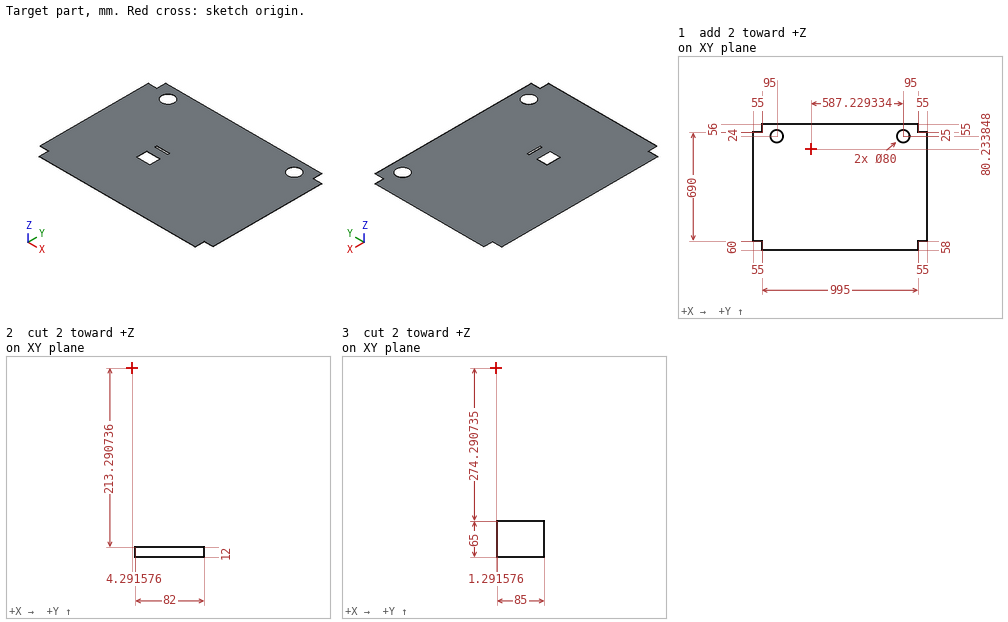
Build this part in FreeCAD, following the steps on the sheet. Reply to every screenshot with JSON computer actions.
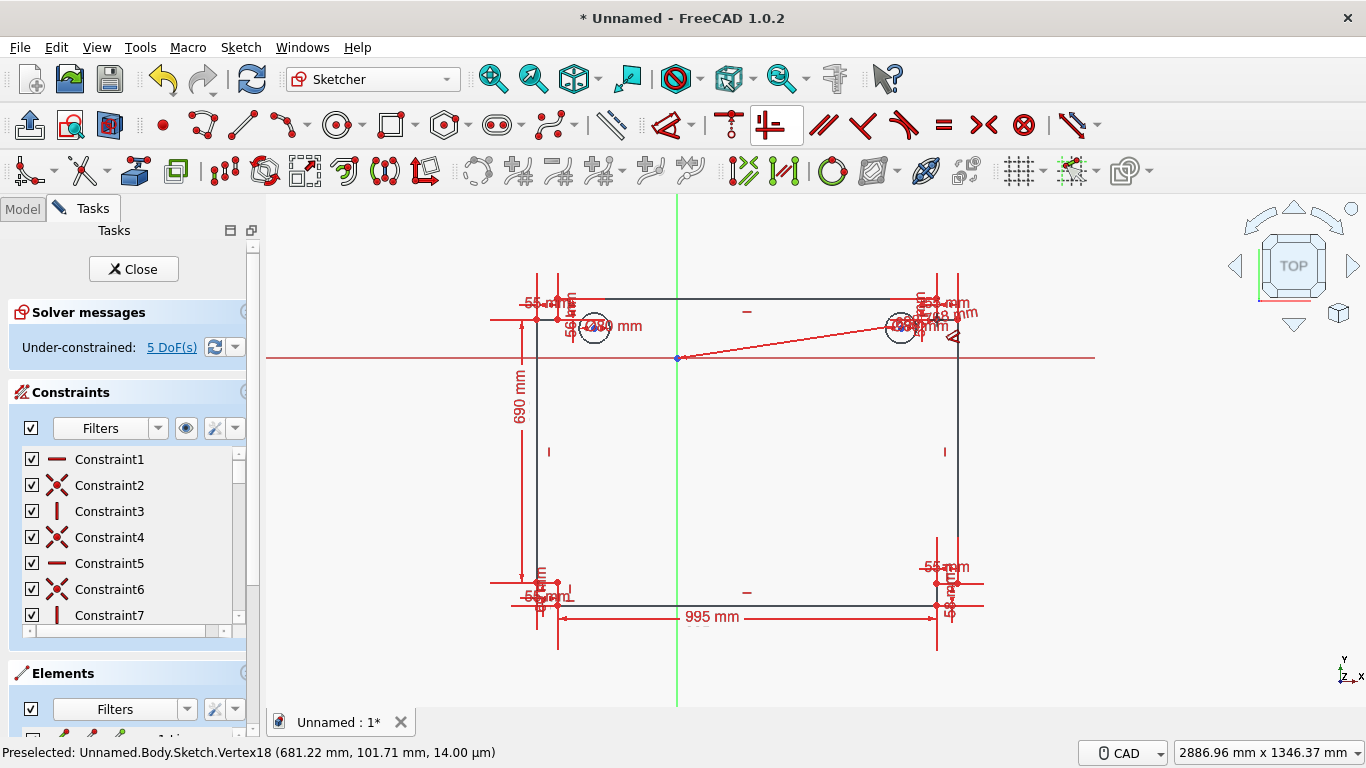
{"action": "left_click", "coordinate": [901, 328]}
{"action": "left_click", "coordinate": [919, 262]}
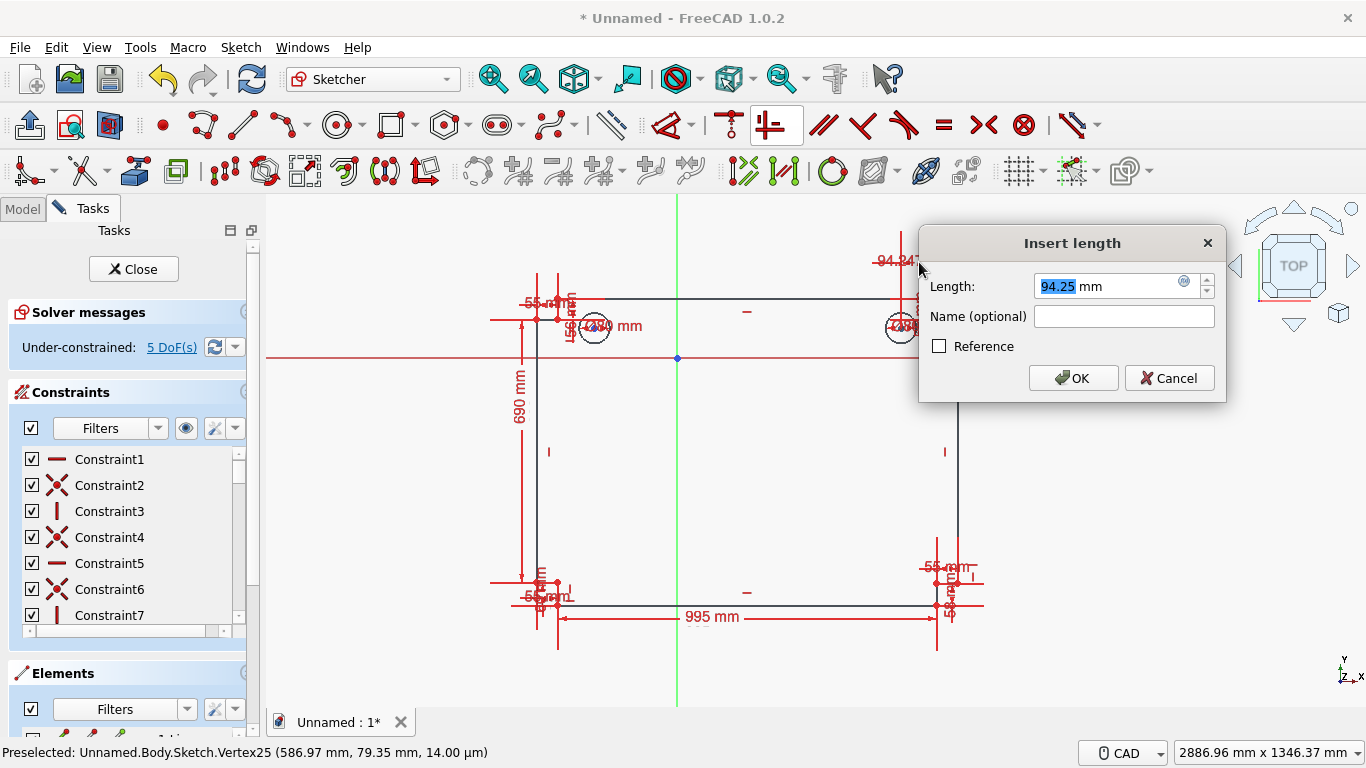
{"action": "type", "text": "95"}
{"action": "key", "text": "Return"}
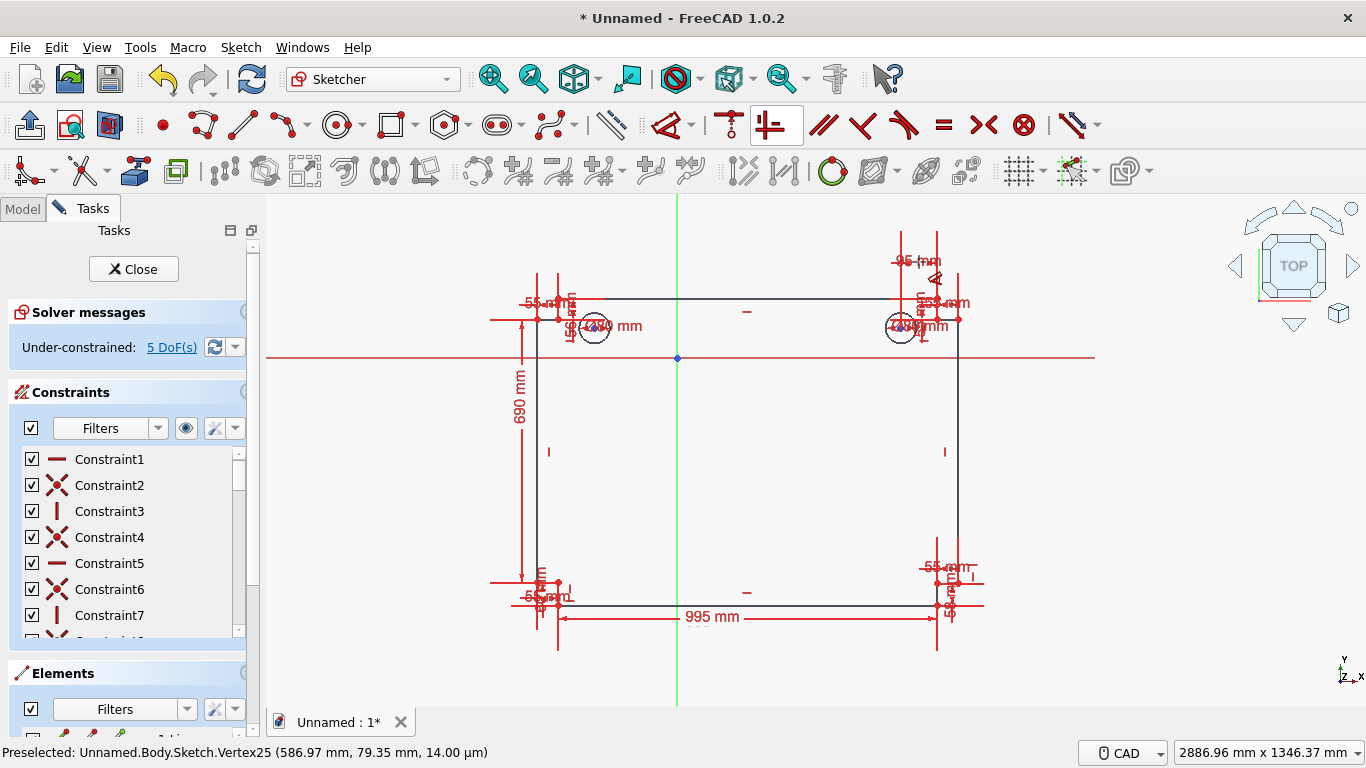
{"action": "scroll", "coordinate": [937, 320], "scroll_direction": "up", "scroll_amount": 8}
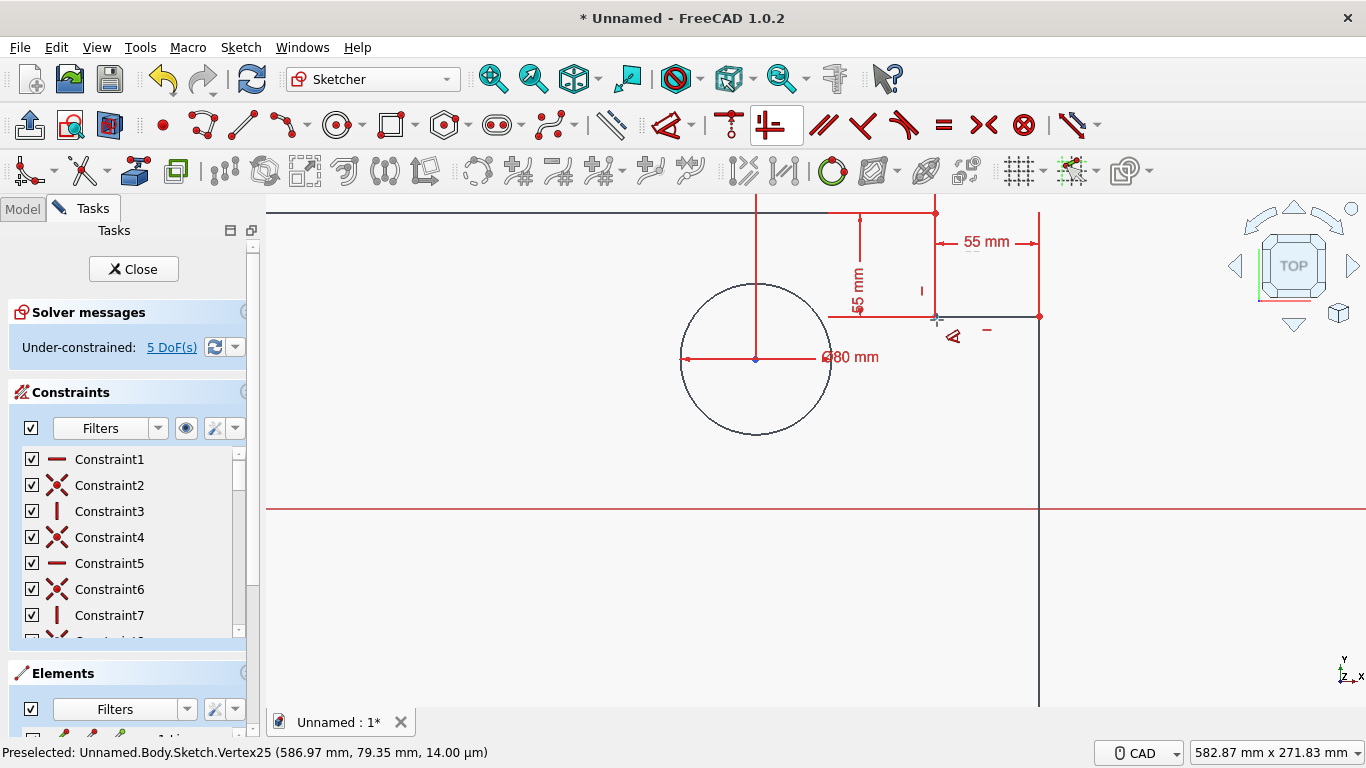
{"action": "left_click", "coordinate": [935, 317]}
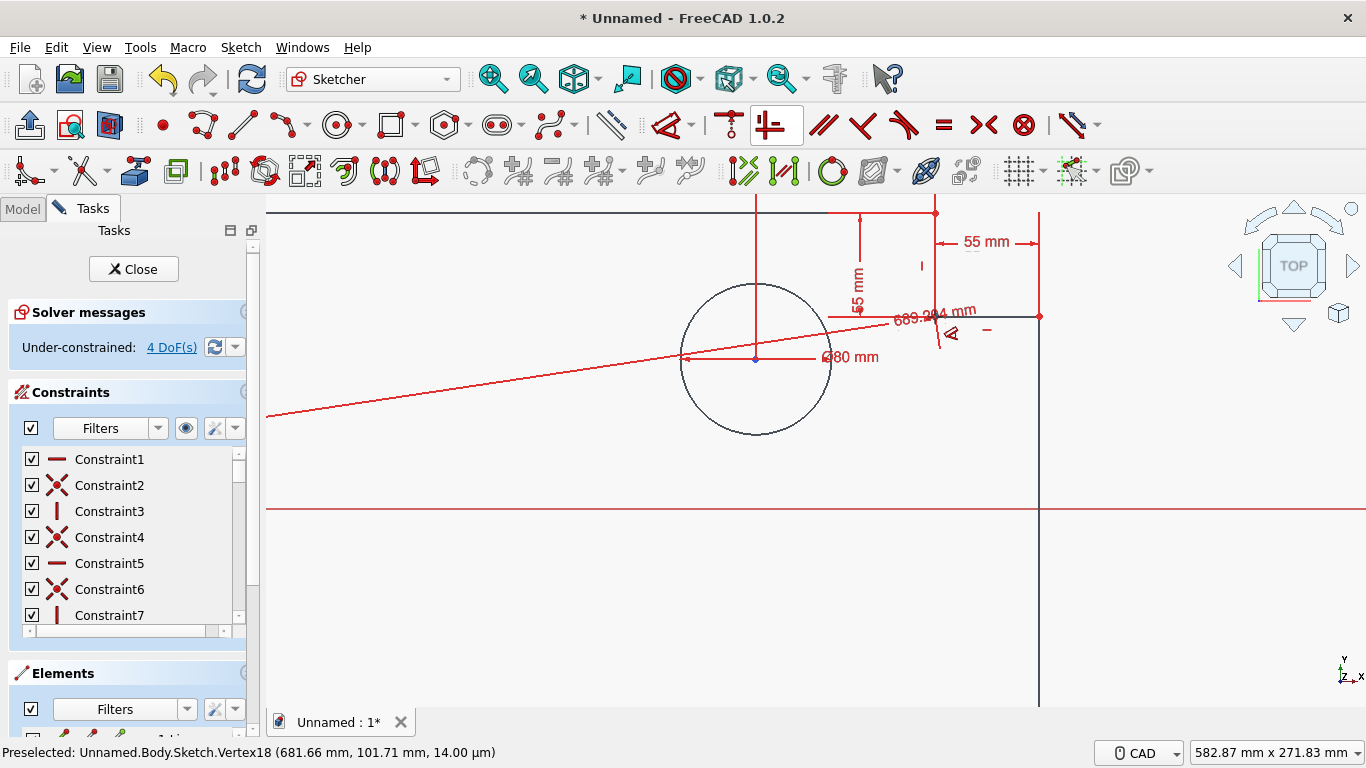
{"action": "left_click", "coordinate": [756, 359]}
{"action": "left_click", "coordinate": [969, 338]}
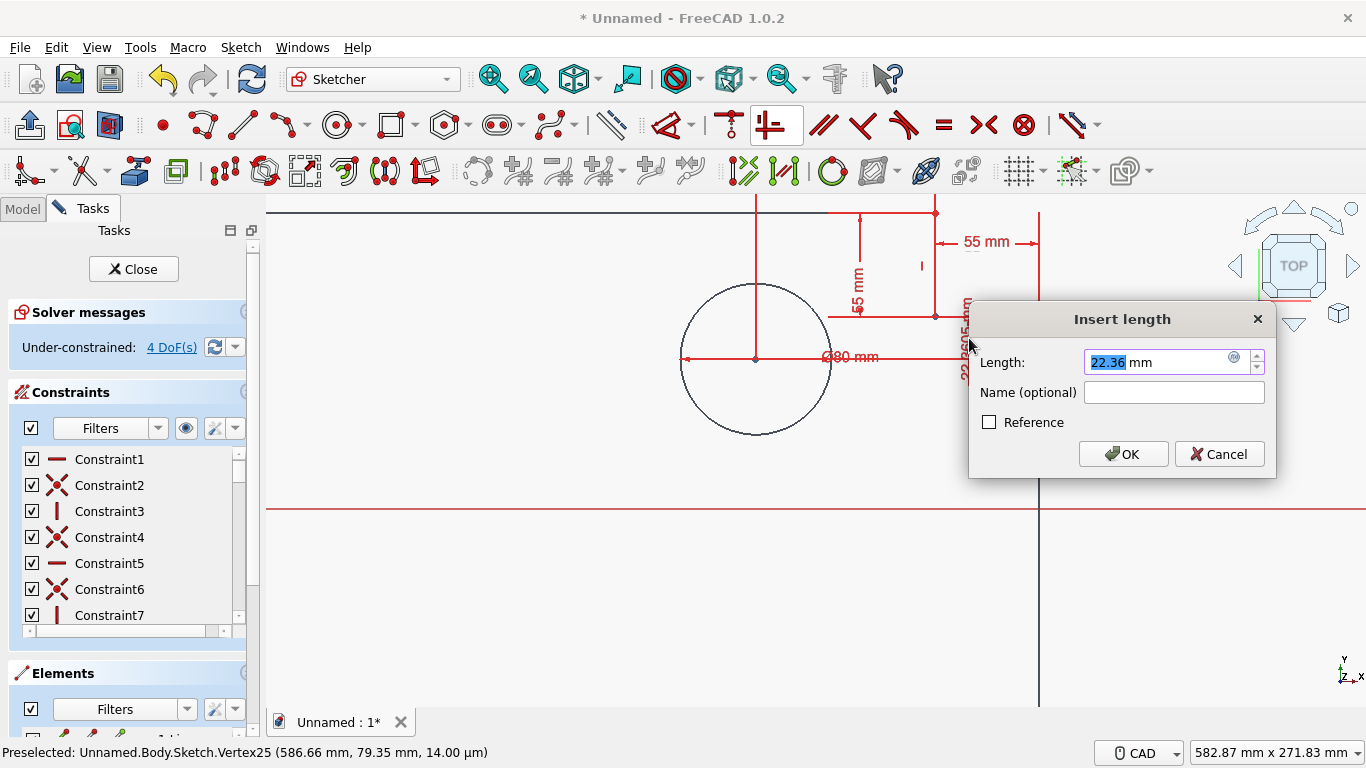
{"action": "type", "text": "25"}
{"action": "key", "text": "Return"}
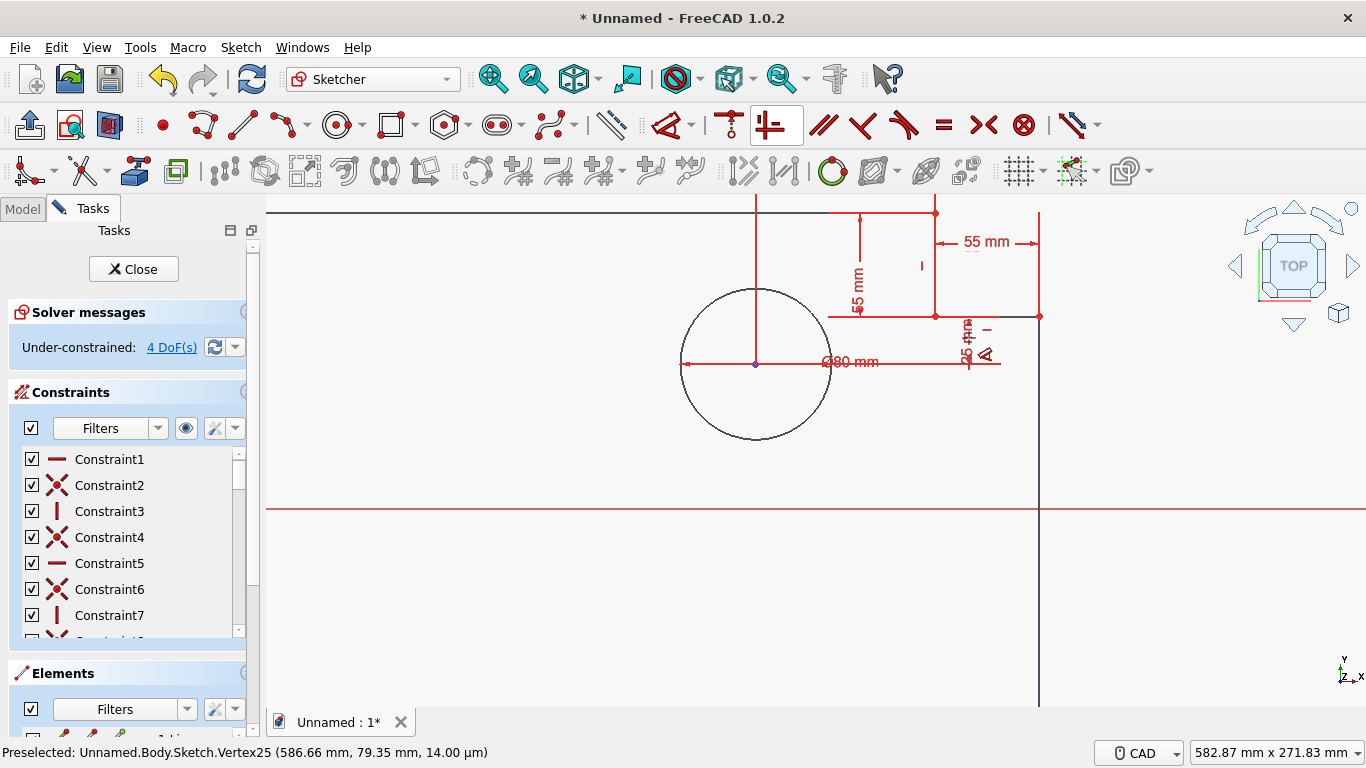
{"action": "scroll", "coordinate": [937, 320], "scroll_direction": "down", "scroll_amount": 8}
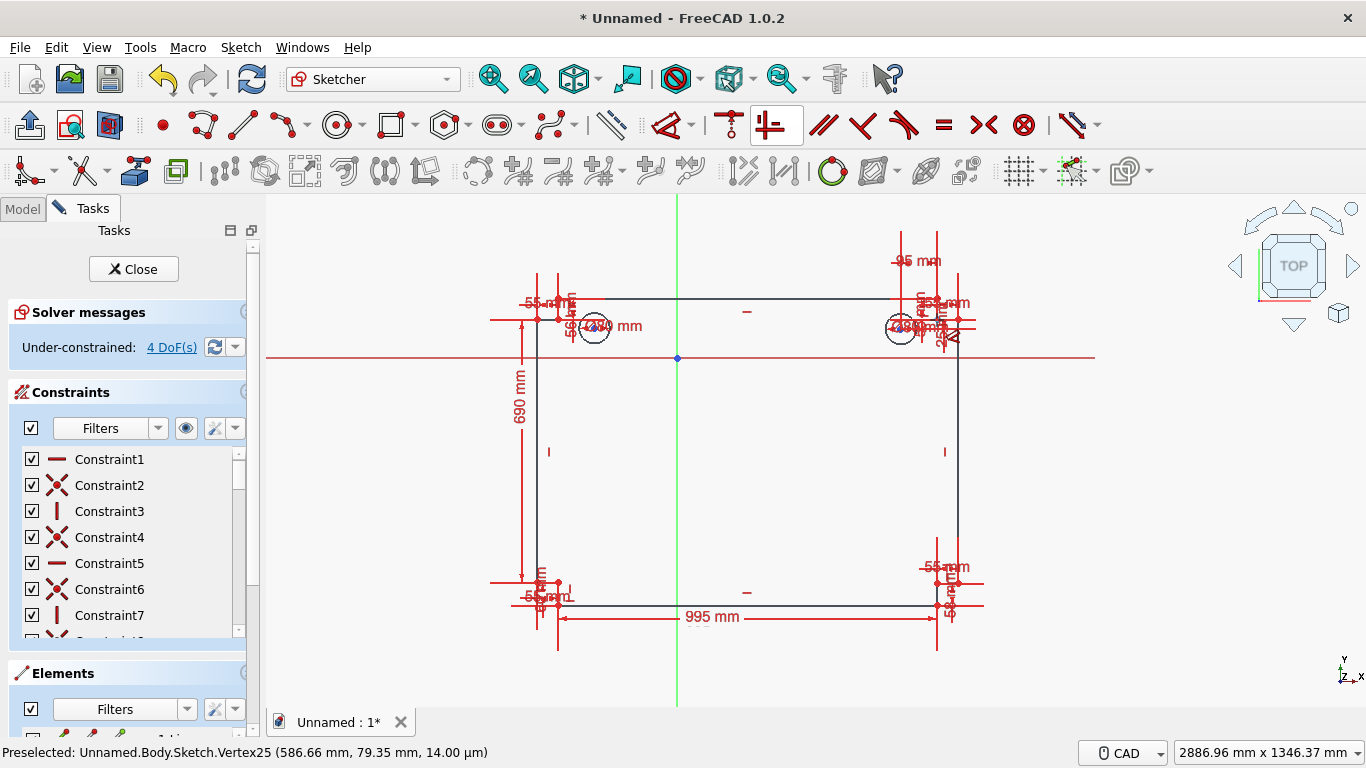
{"action": "left_click", "coordinate": [558, 320]}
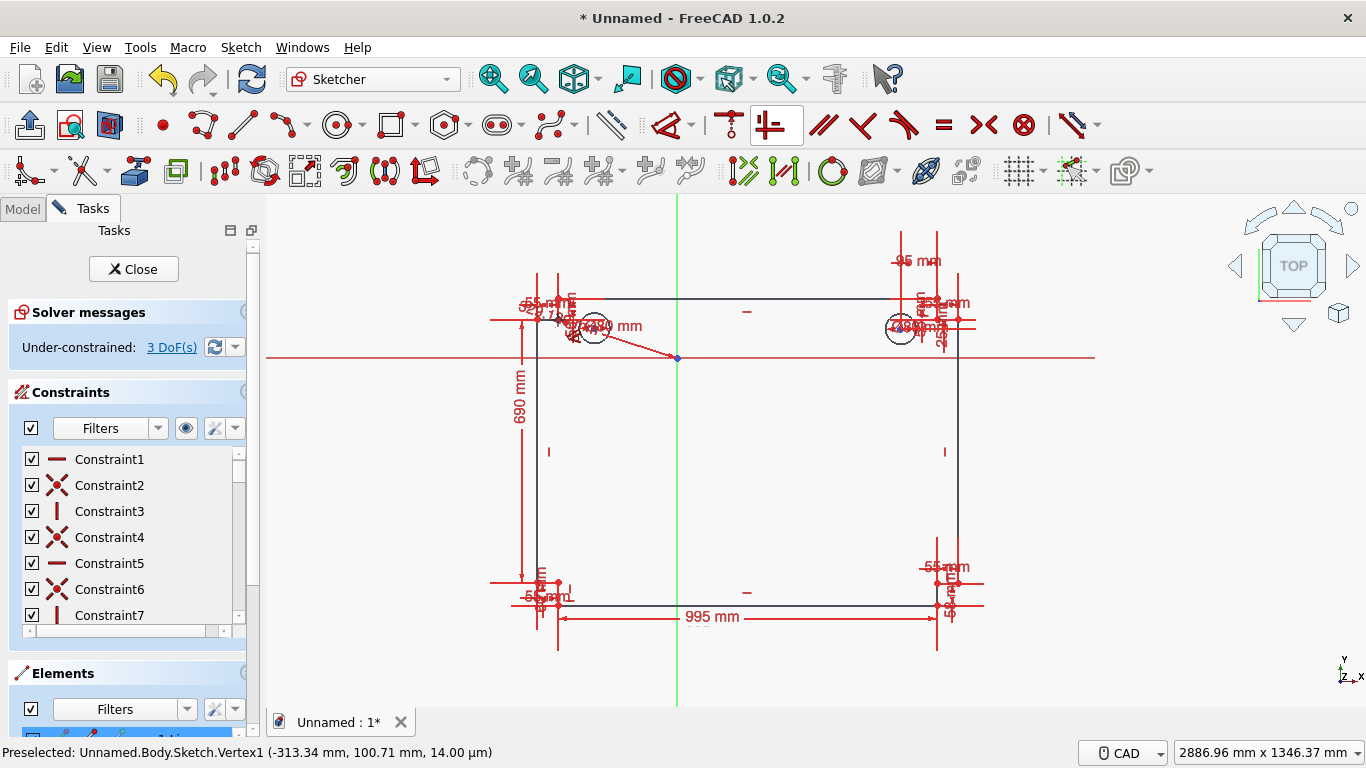
{"action": "left_click", "coordinate": [594, 328]}
{"action": "left_click", "coordinate": [576, 262]}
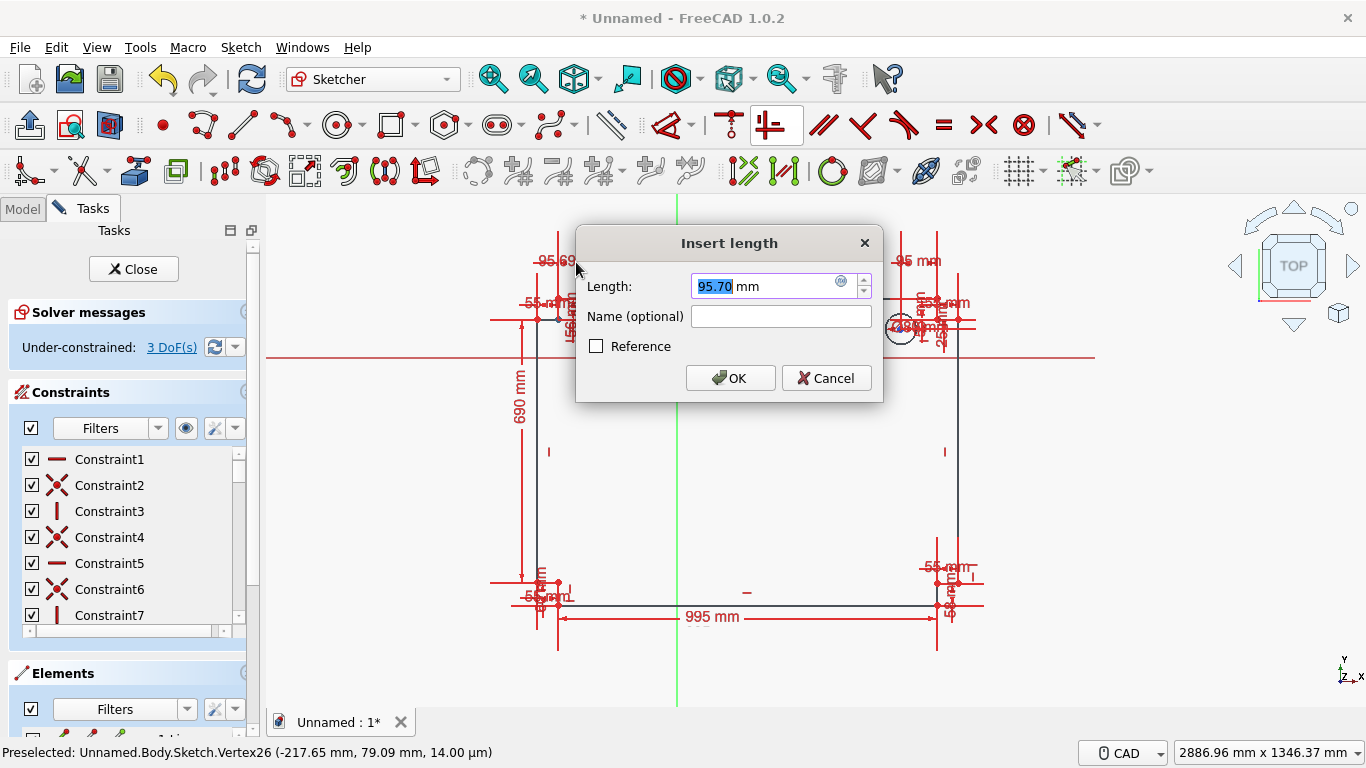
{"action": "type", "text": "95"}
{"action": "key", "text": "Return"}